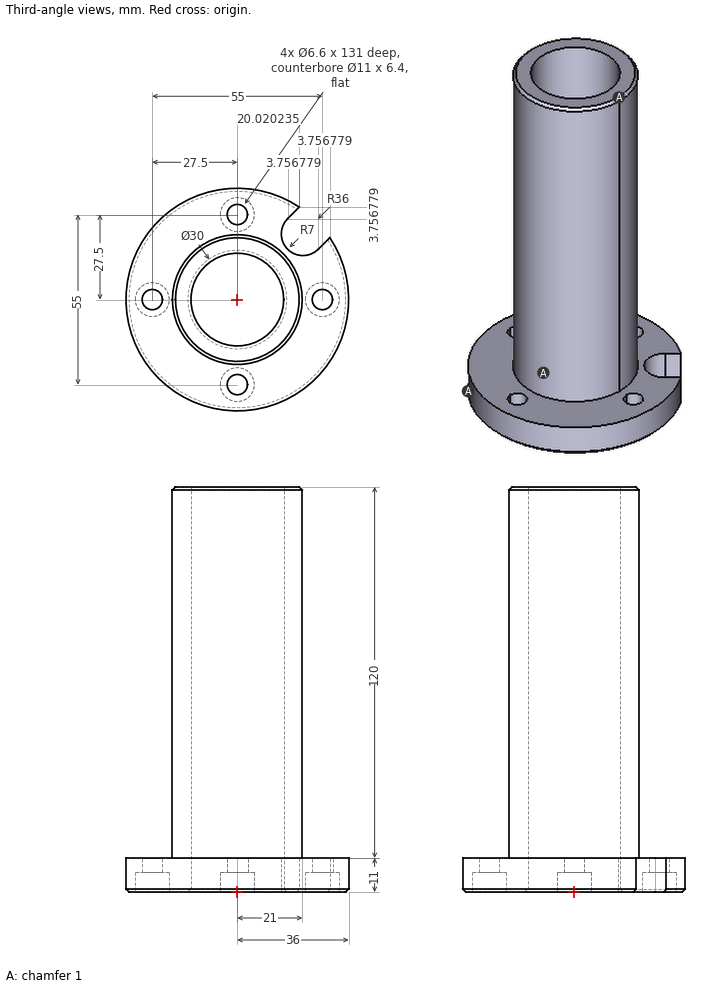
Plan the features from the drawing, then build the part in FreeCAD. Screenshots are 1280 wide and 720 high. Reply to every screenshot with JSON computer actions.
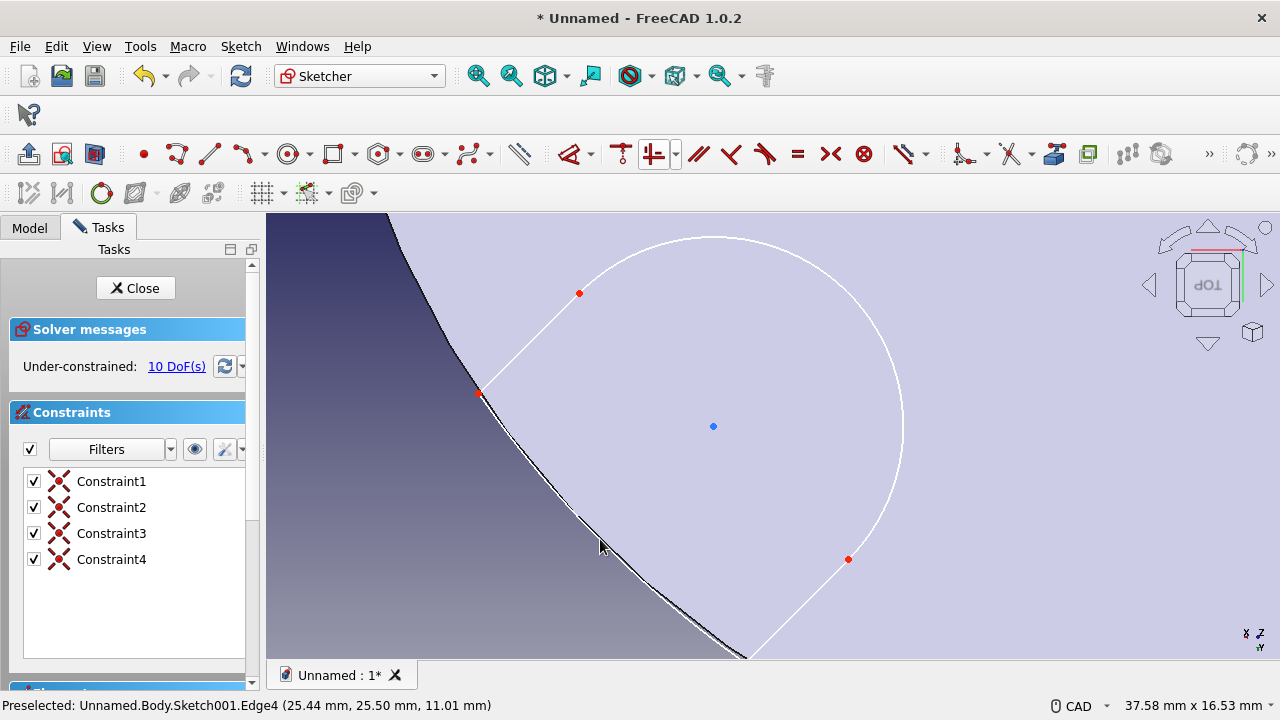
{"action": "left_click", "coordinate": [818, 590]}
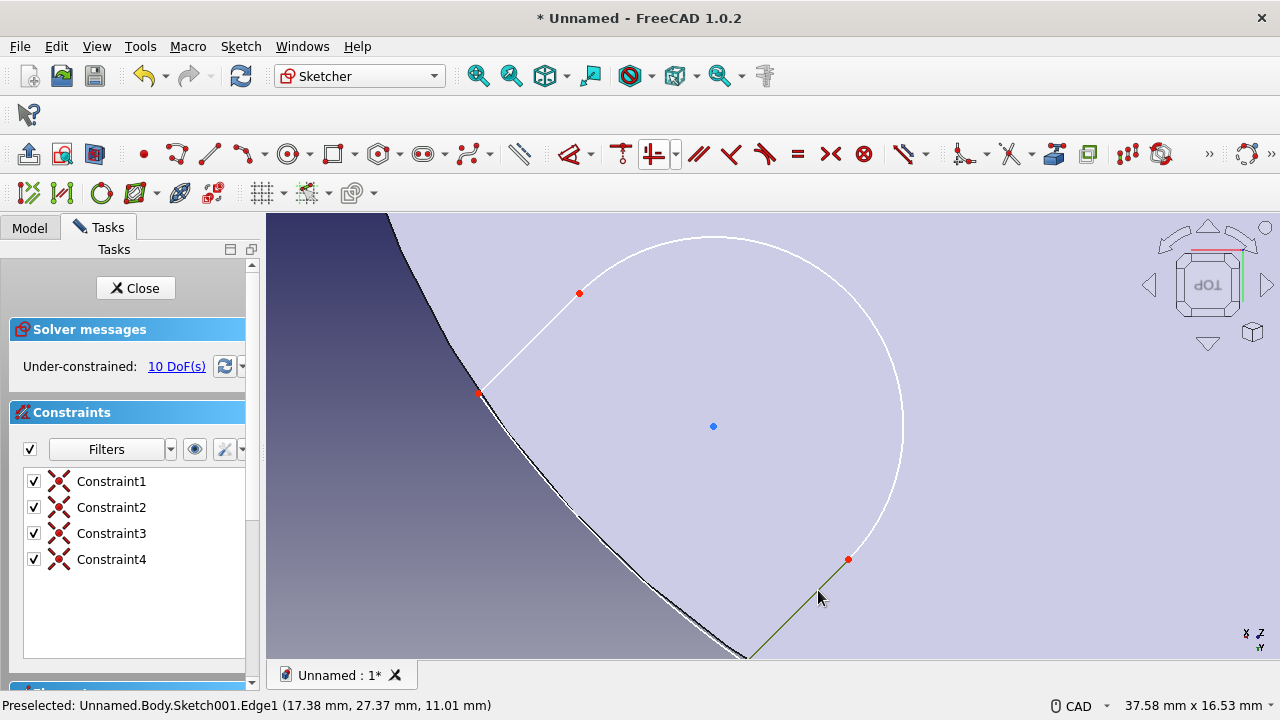
{"action": "left_click", "coordinate": [901, 396]}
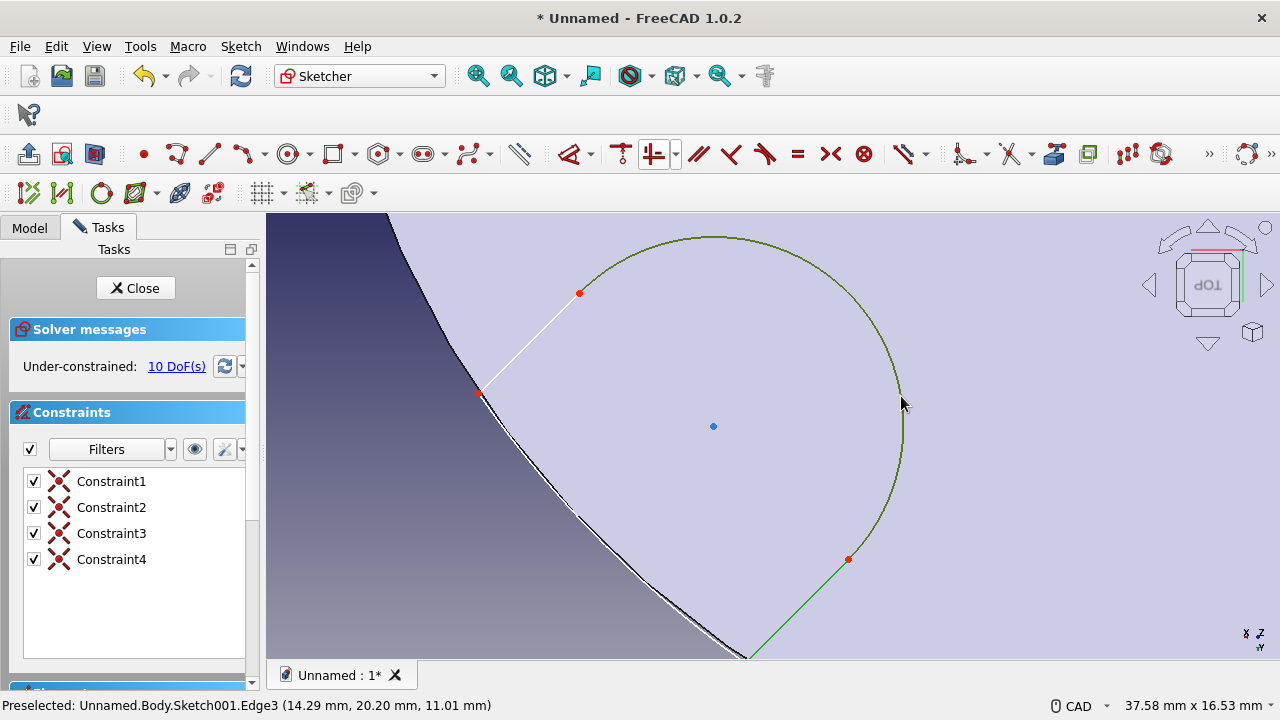
{"action": "left_click", "coordinate": [765, 154]}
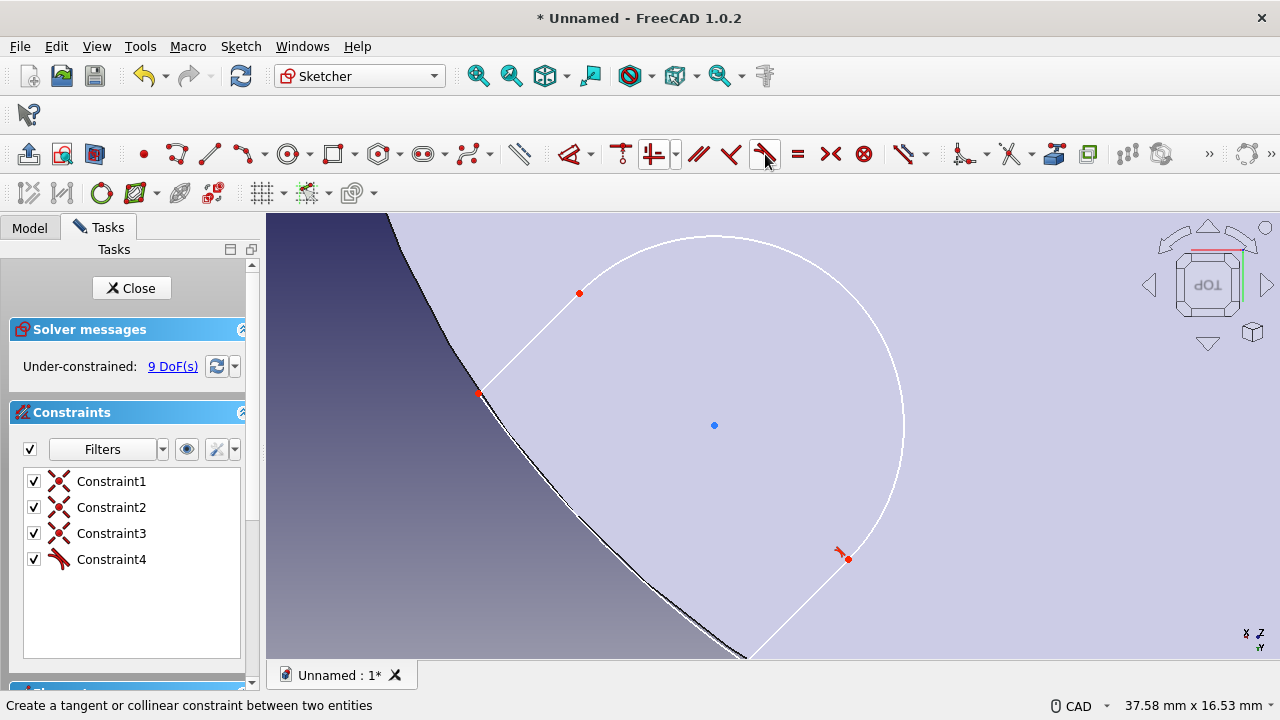
{"action": "left_click", "coordinate": [549, 323]}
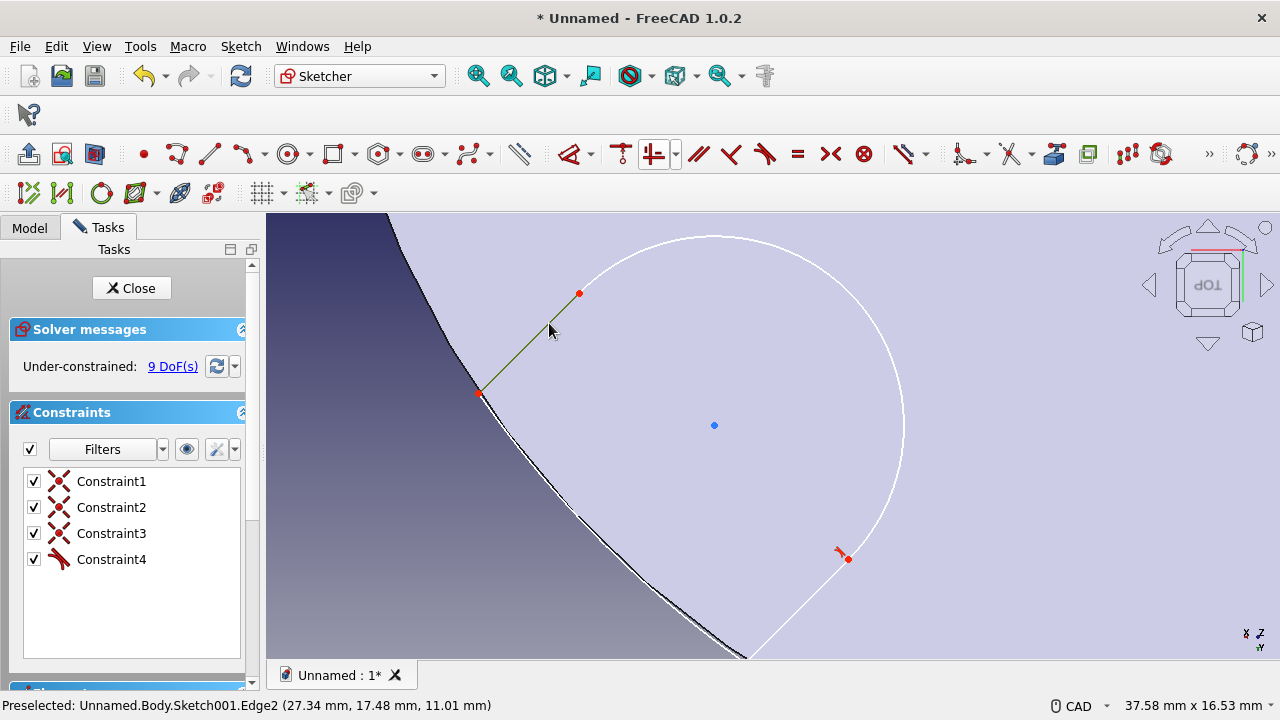
{"action": "left_click", "coordinate": [902, 395]}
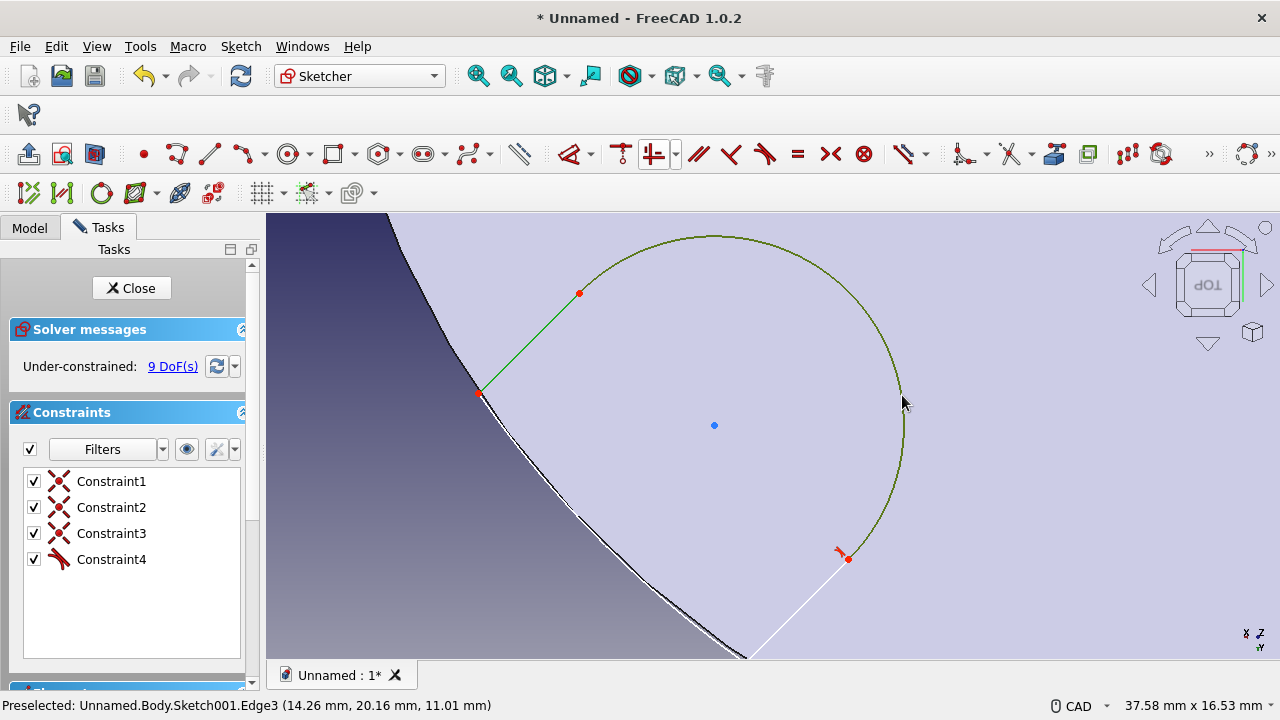
{"action": "left_click", "coordinate": [765, 154]}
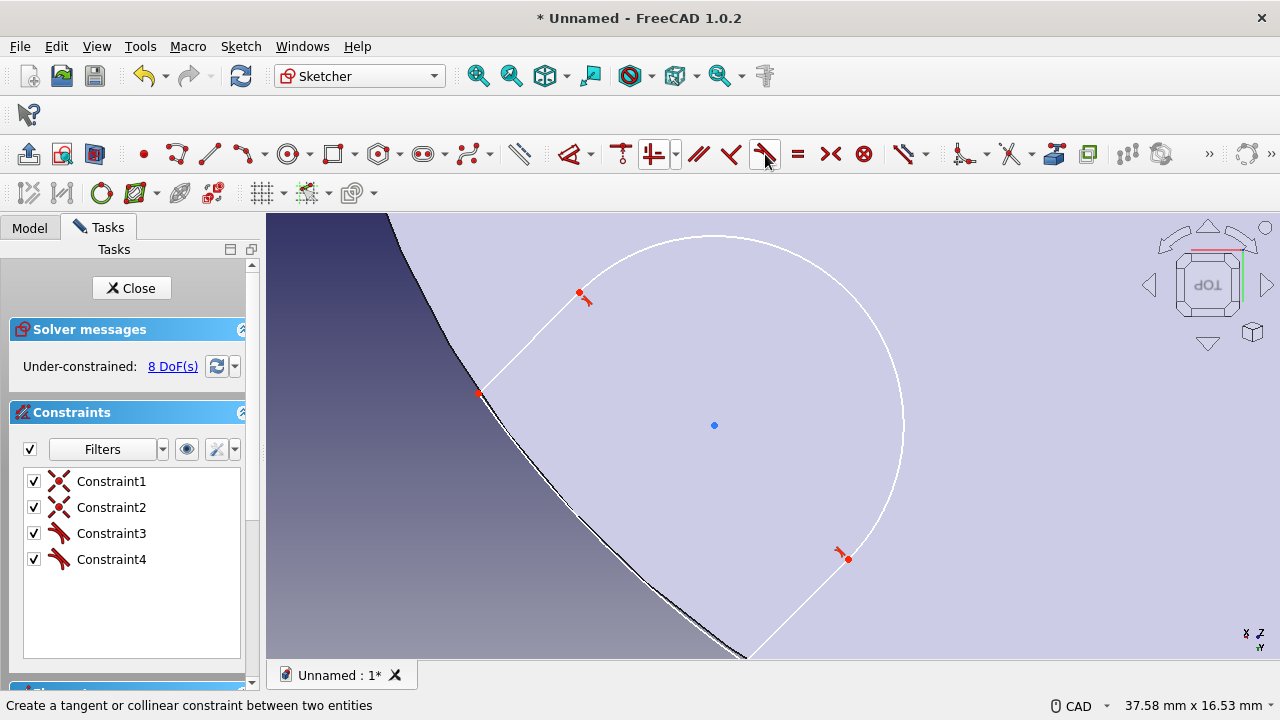
{"action": "scroll", "coordinate": [601, 541], "scroll_direction": "down", "scroll_amount": 5}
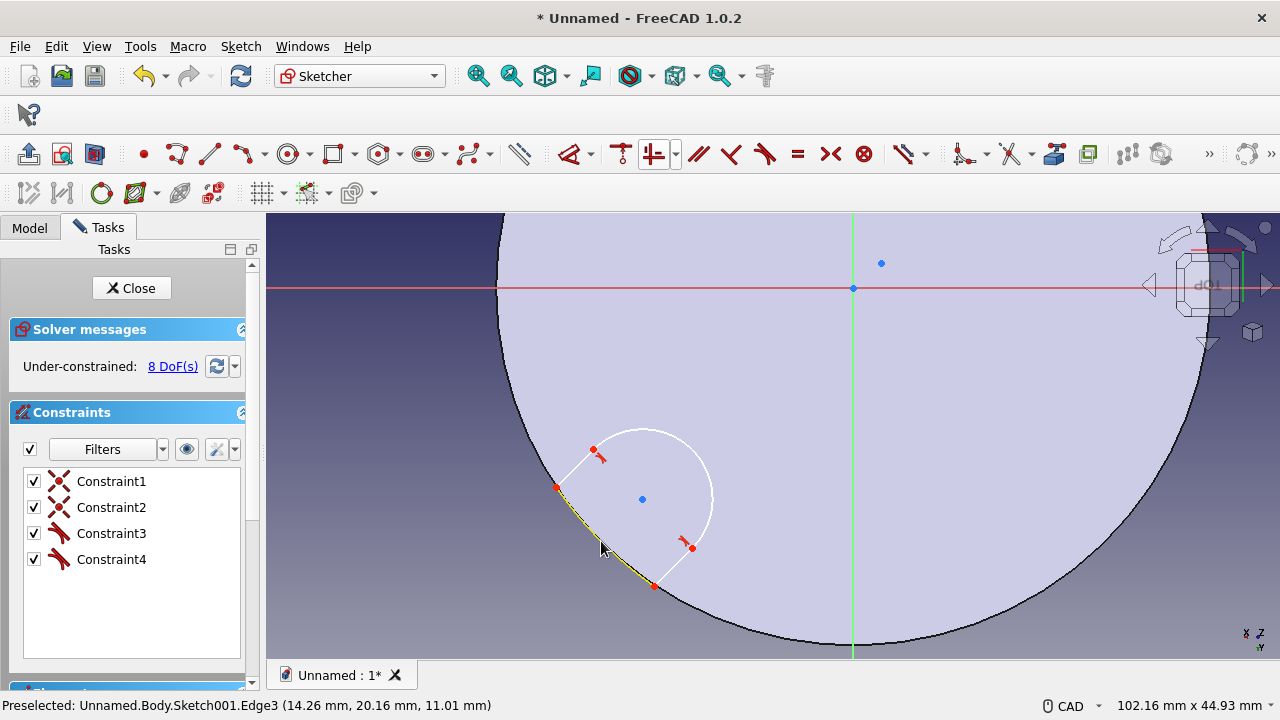
{"action": "left_click_drag", "start_coordinate": [843, 253], "coordinate": [892, 298]}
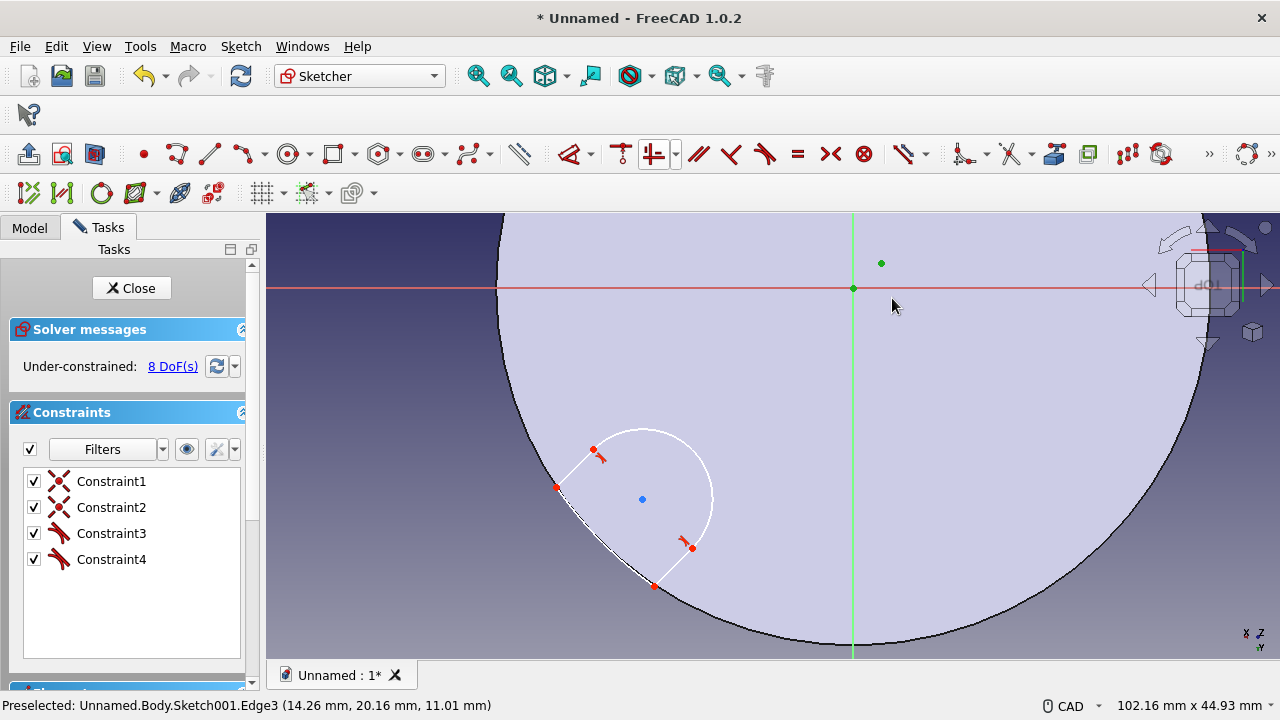
{"action": "left_click", "coordinate": [621, 154]}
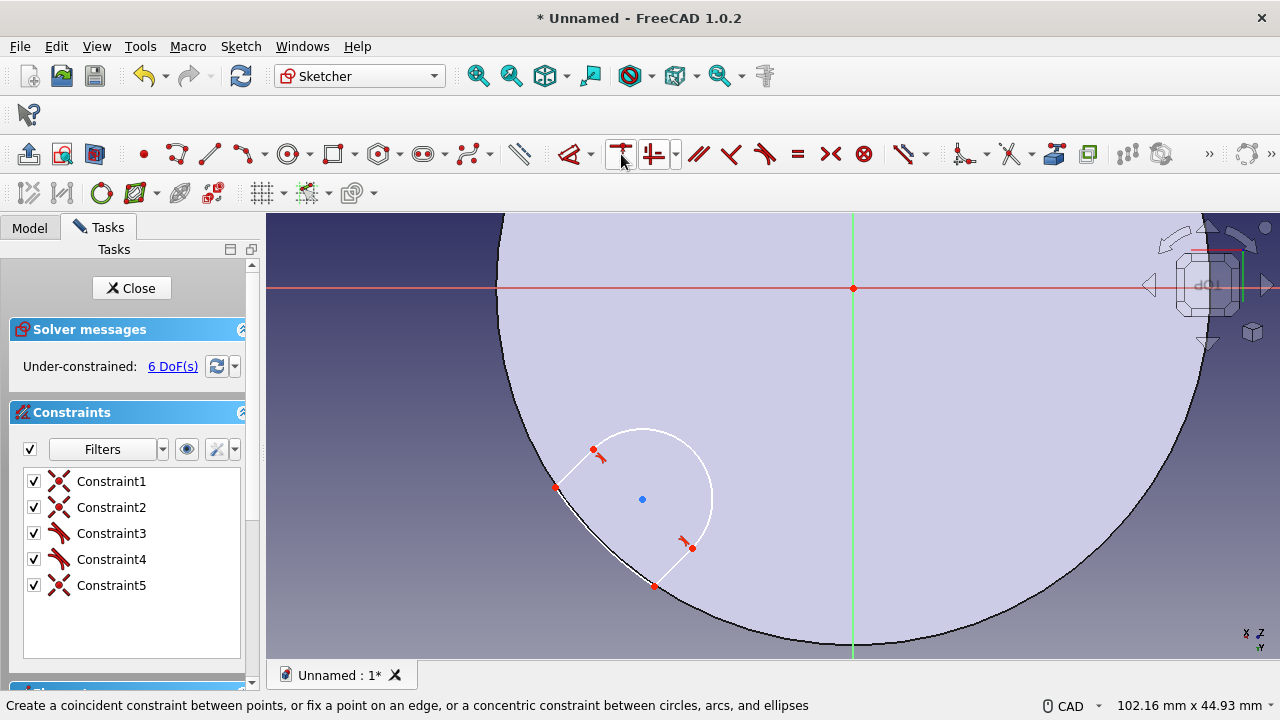
{"action": "left_click", "coordinate": [568, 154]}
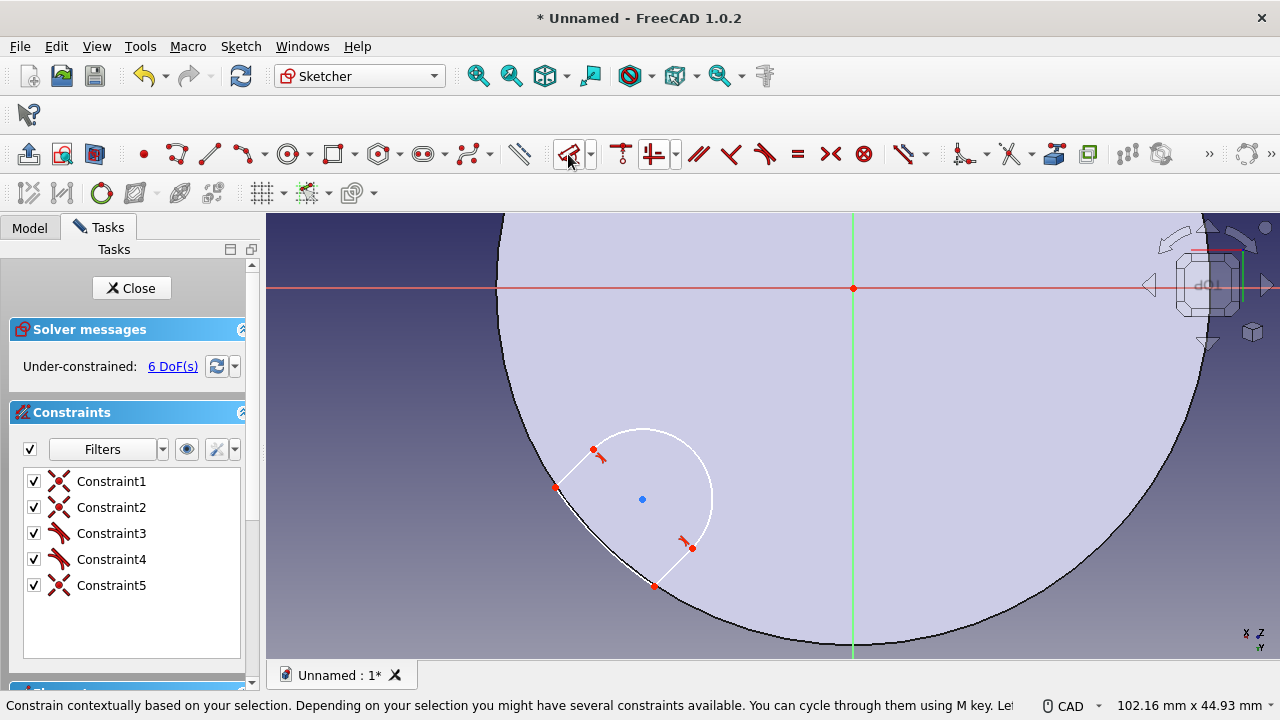
{"action": "left_click", "coordinate": [711, 488]}
{"action": "left_click", "coordinate": [743, 483]}